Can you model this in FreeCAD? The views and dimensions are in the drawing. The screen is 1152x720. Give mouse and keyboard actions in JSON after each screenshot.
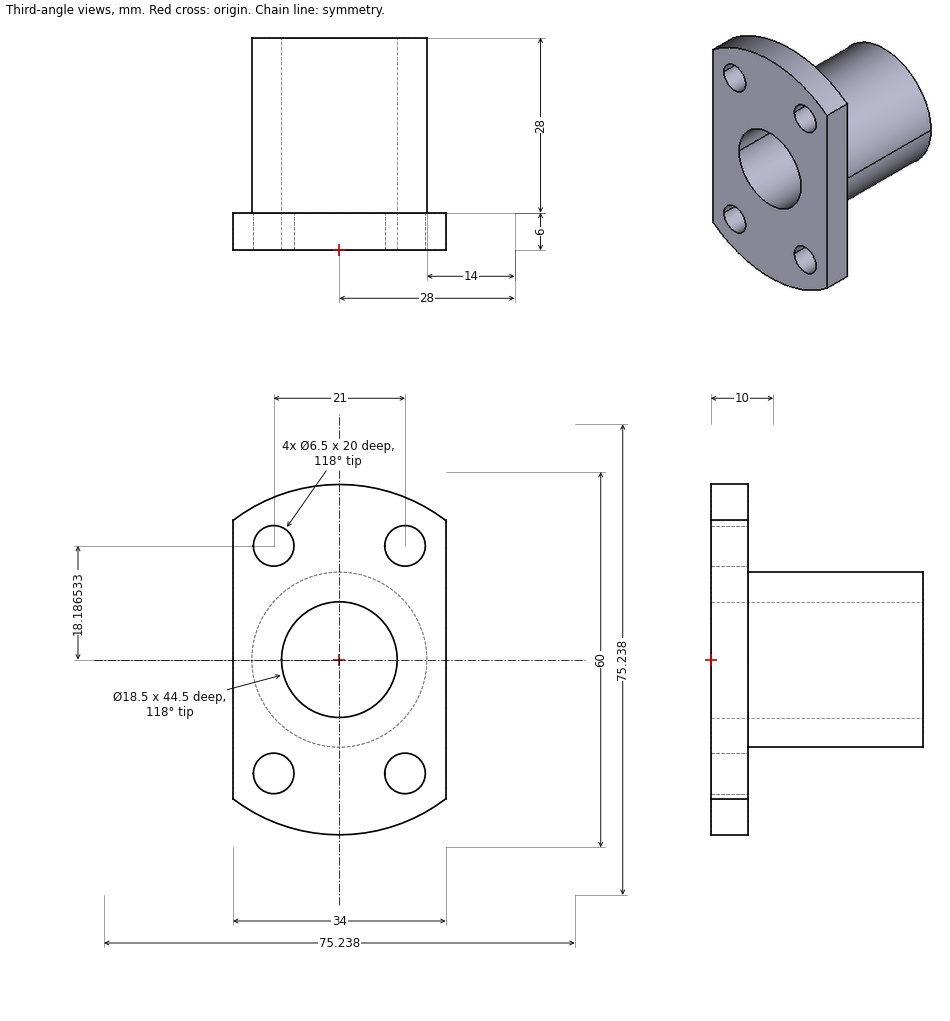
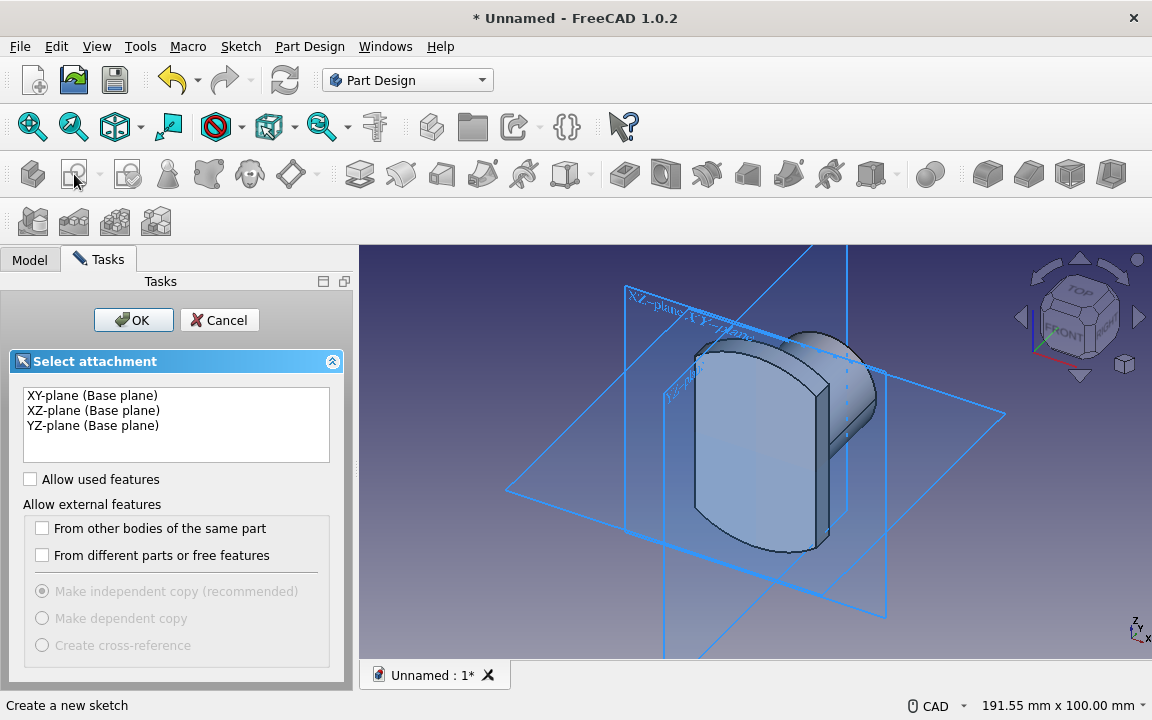
{"action": "left_click", "coordinate": [84, 410]}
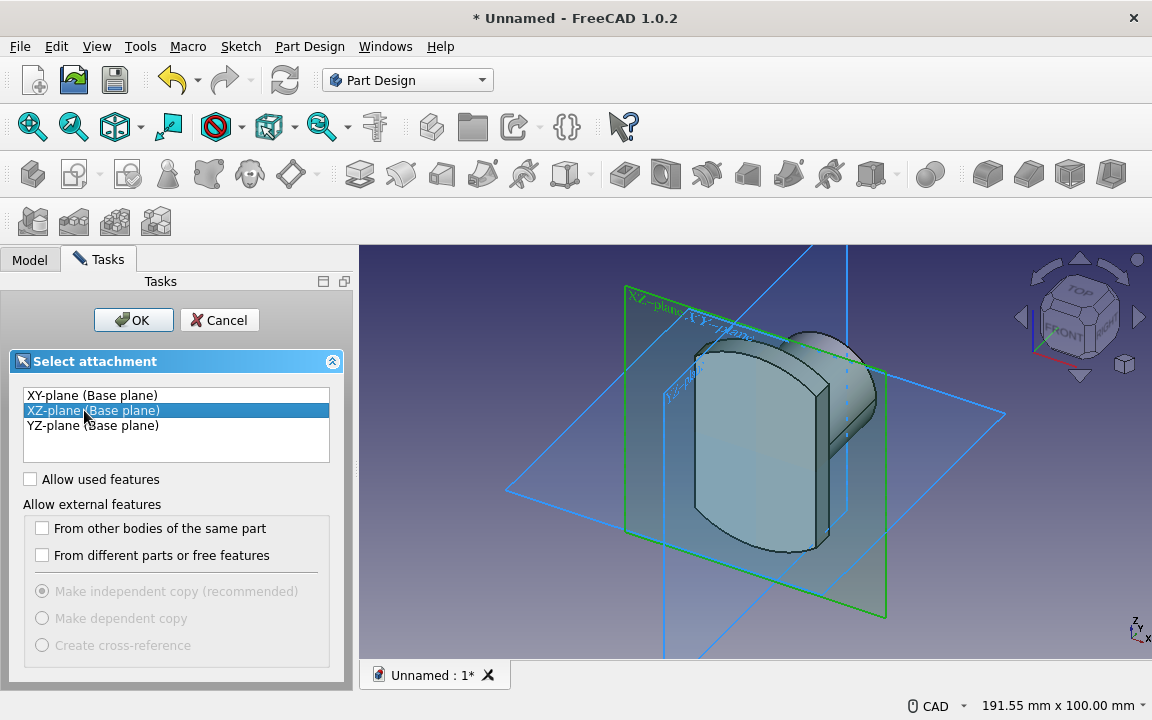
{"action": "left_click", "coordinate": [134, 320]}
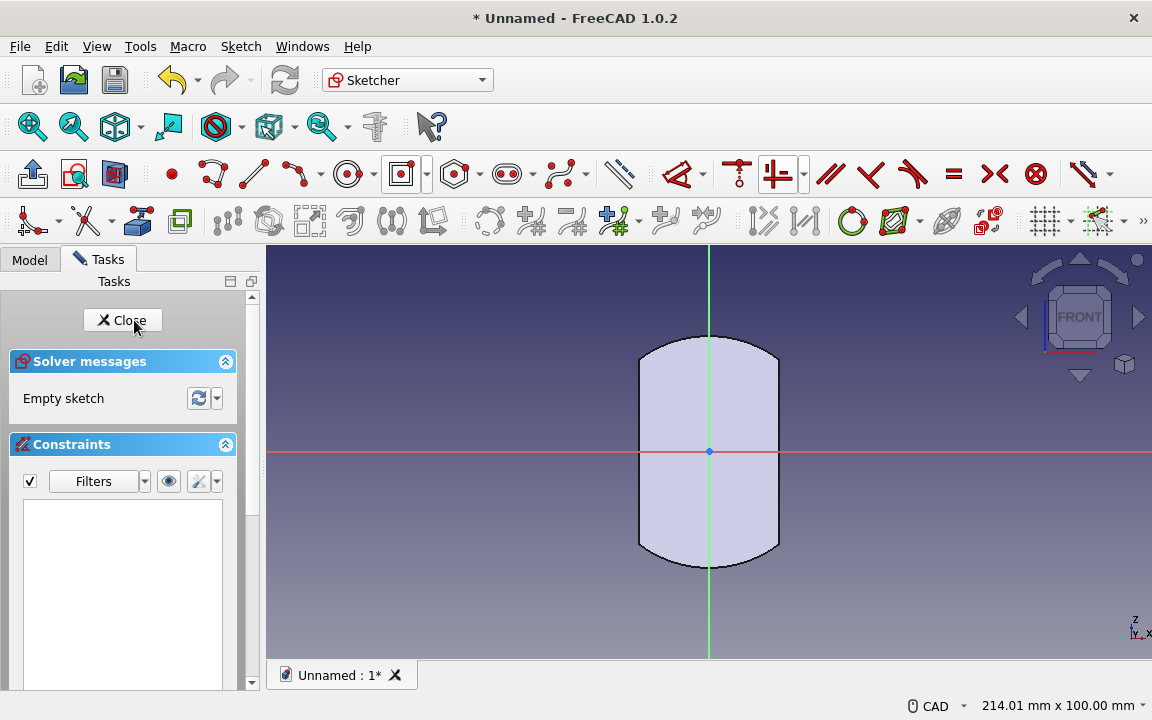
{"action": "scroll", "coordinate": [848, 452], "scroll_direction": "up", "scroll_amount": 2}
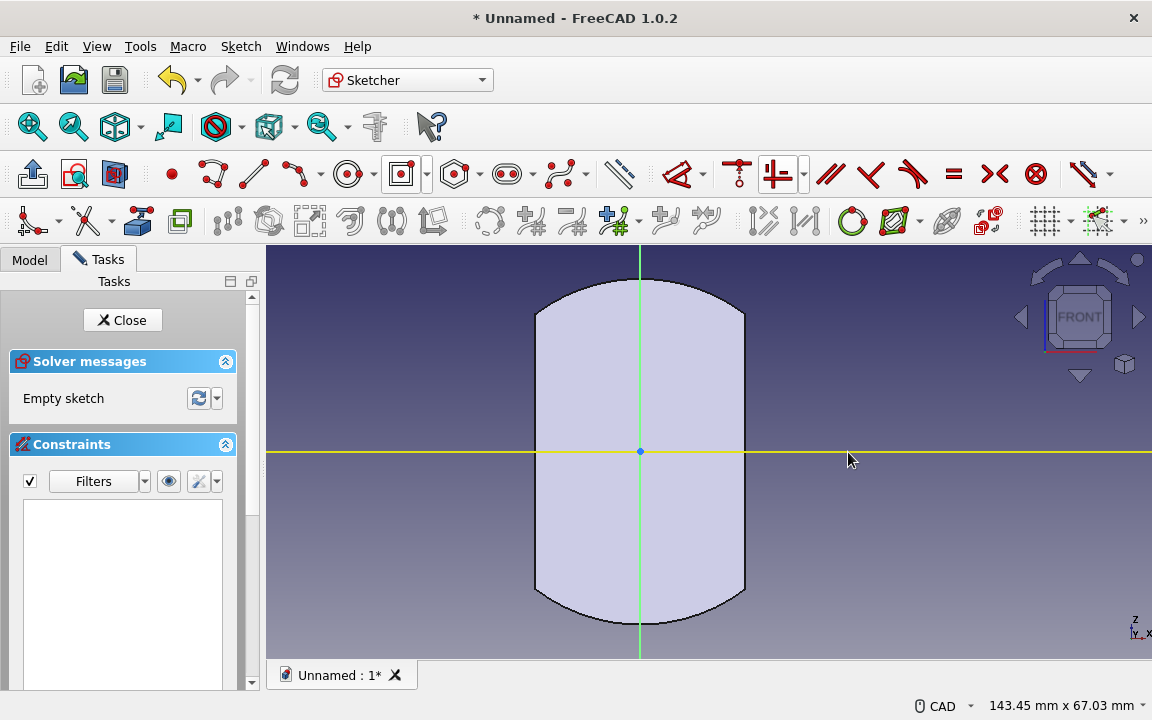
{"action": "left_click", "coordinate": [348, 174]}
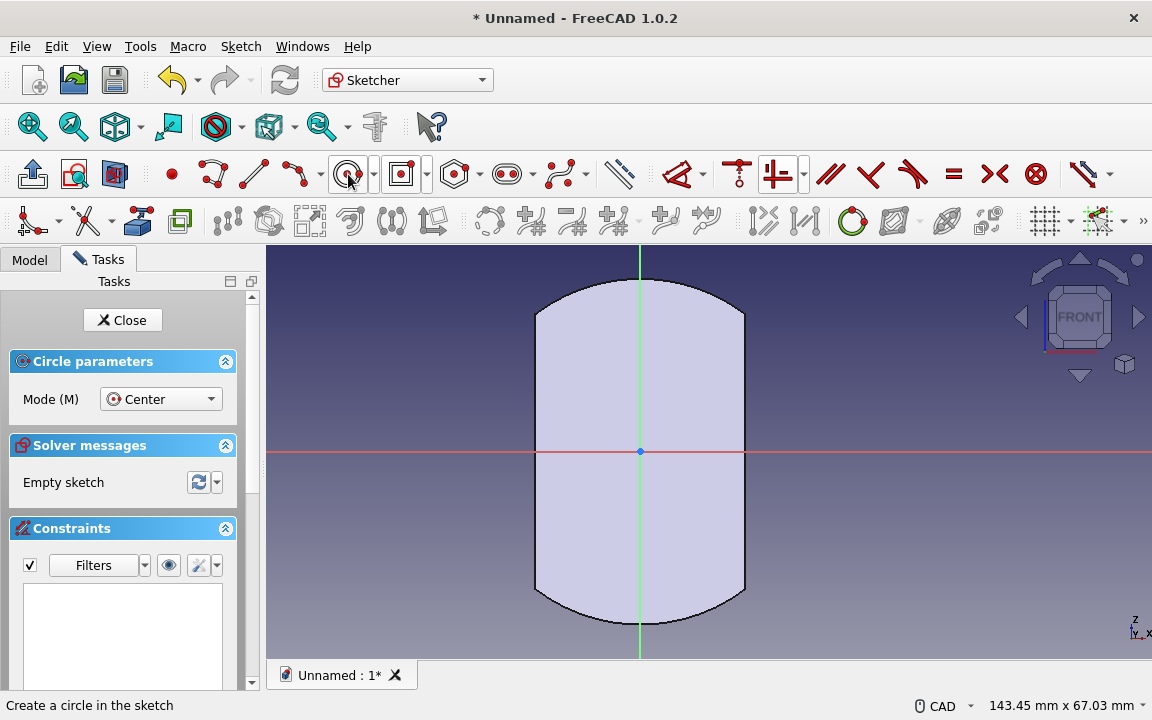
{"action": "left_click", "coordinate": [575, 339]}
{"action": "mouse_move", "coordinate": [590, 325]}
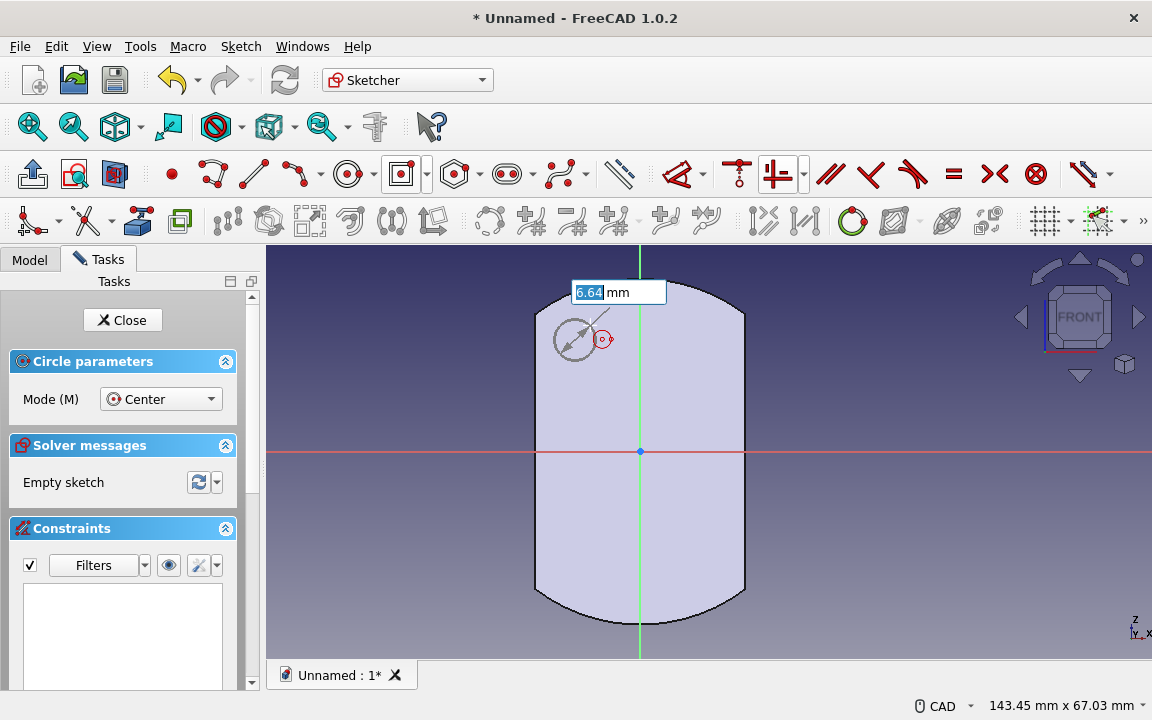
{"action": "type", "text": "6.5"}
{"action": "key", "text": "Return"}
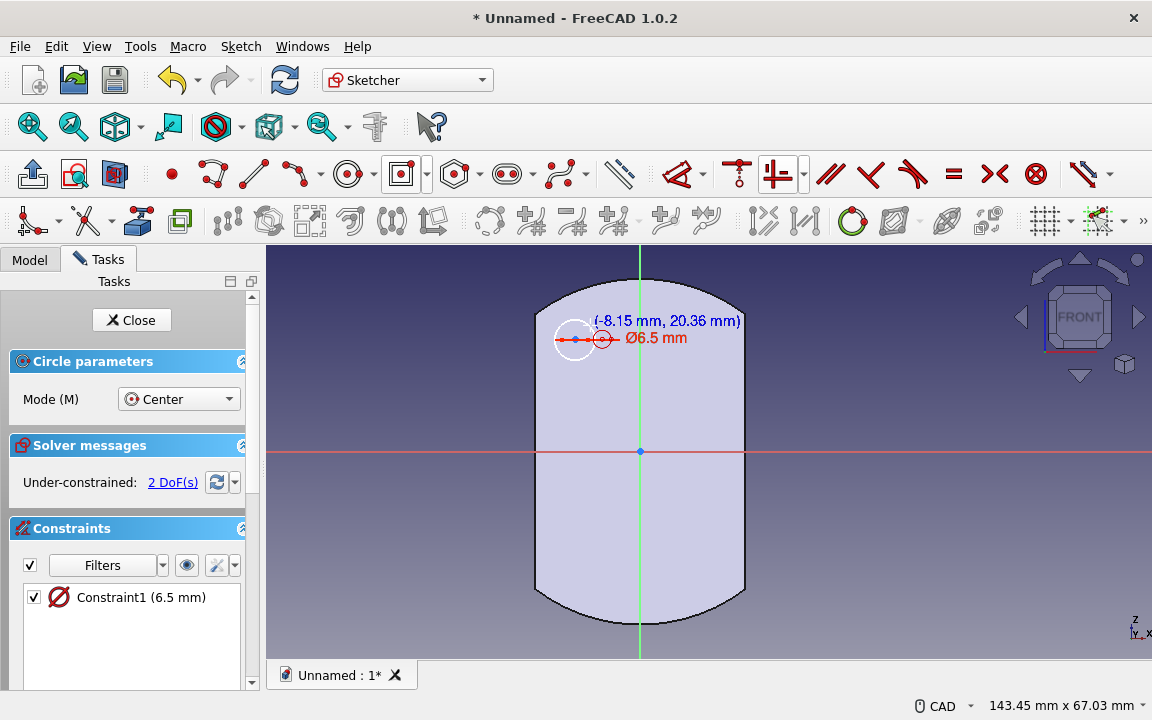
{"action": "left_click", "coordinate": [705, 339]}
{"action": "mouse_move", "coordinate": [719, 325]}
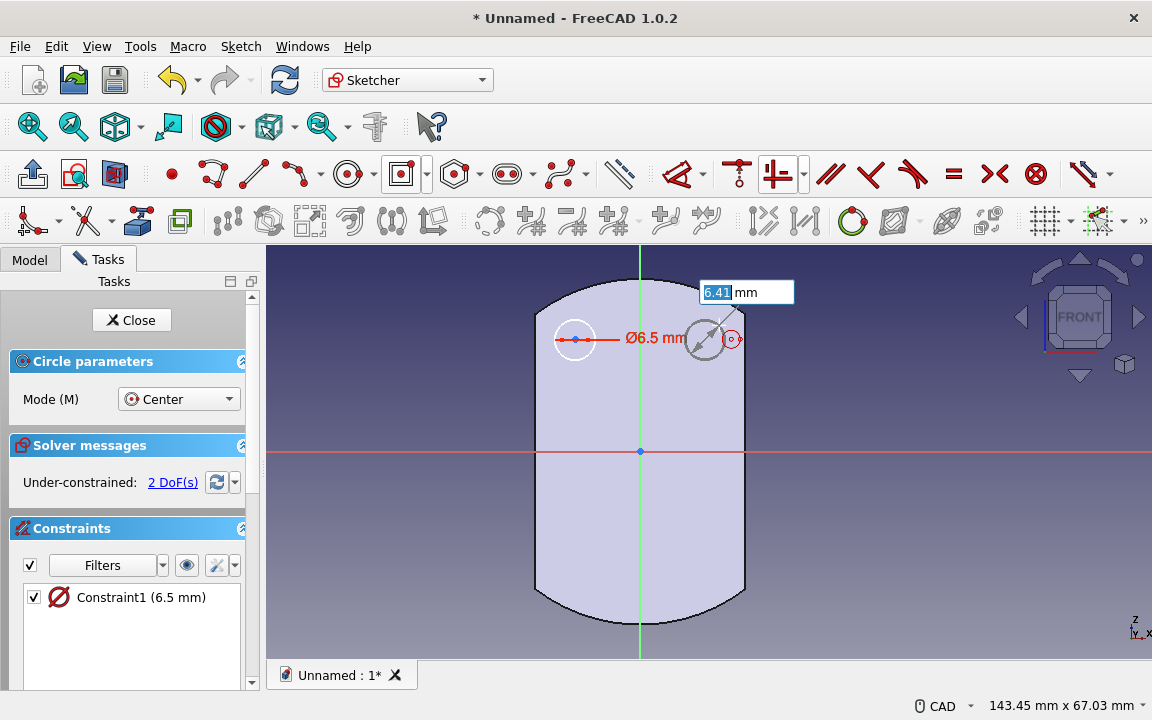
{"action": "type", "text": "6.5"}
{"action": "key", "text": "Return"}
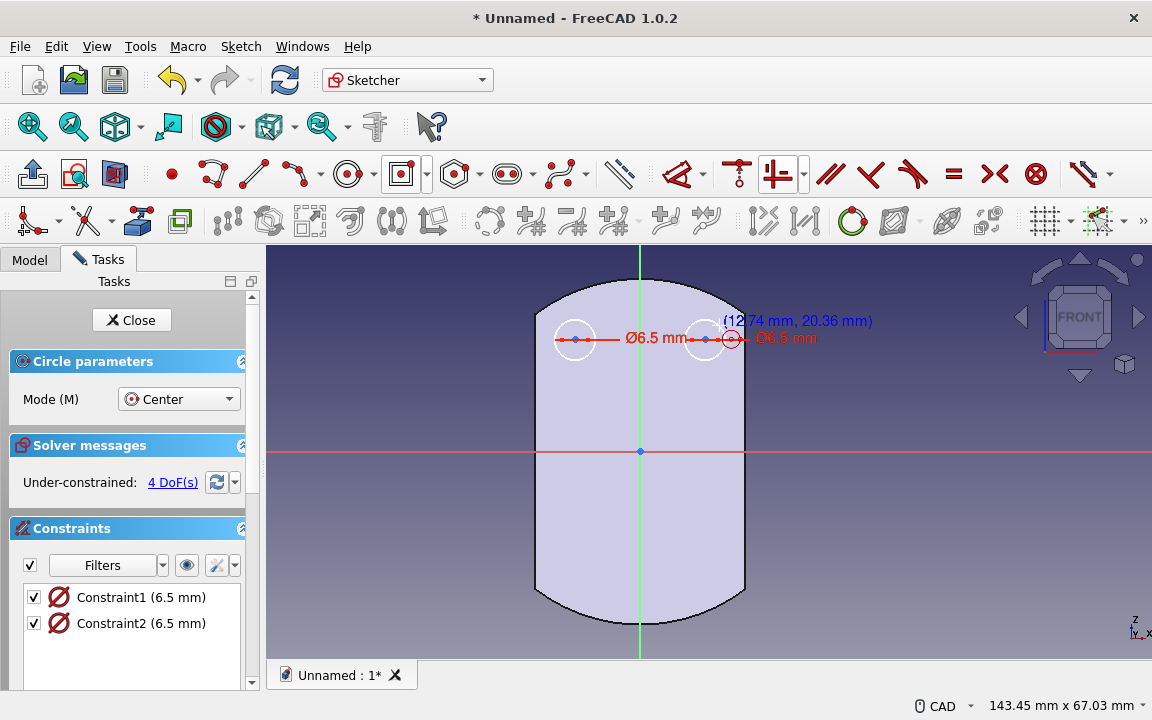
{"action": "left_click", "coordinate": [575, 564]}
{"action": "mouse_move", "coordinate": [590, 550]}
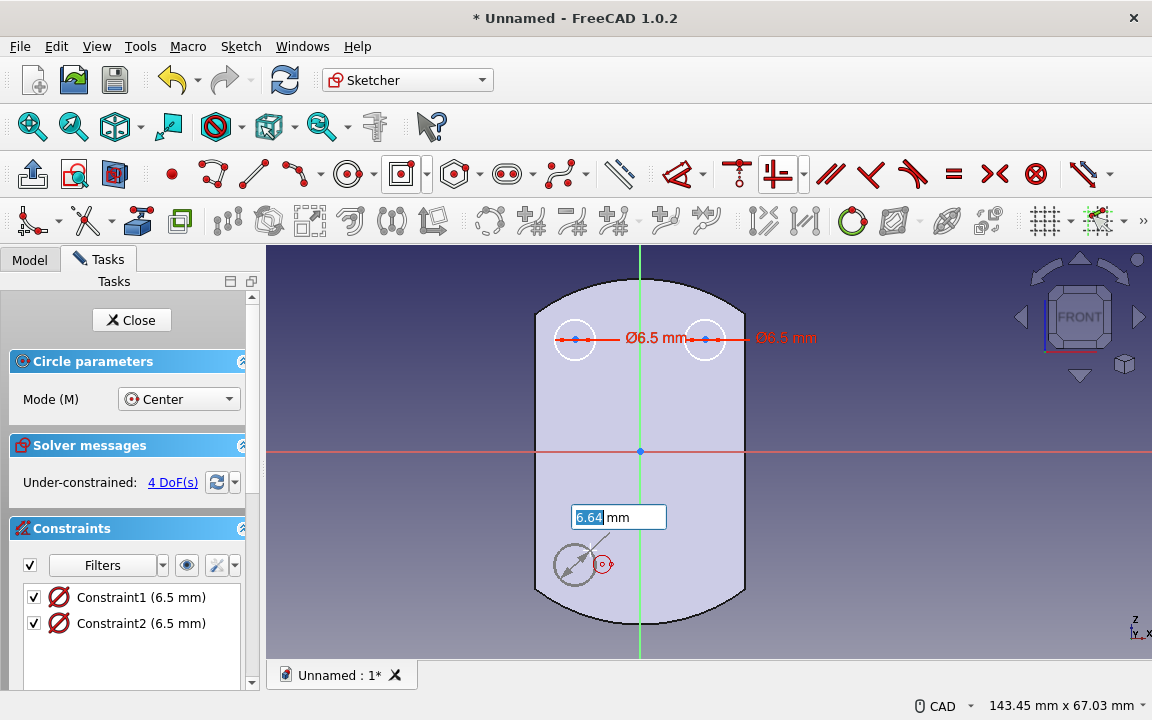
{"action": "type", "text": "6.5"}
{"action": "key", "text": "Return"}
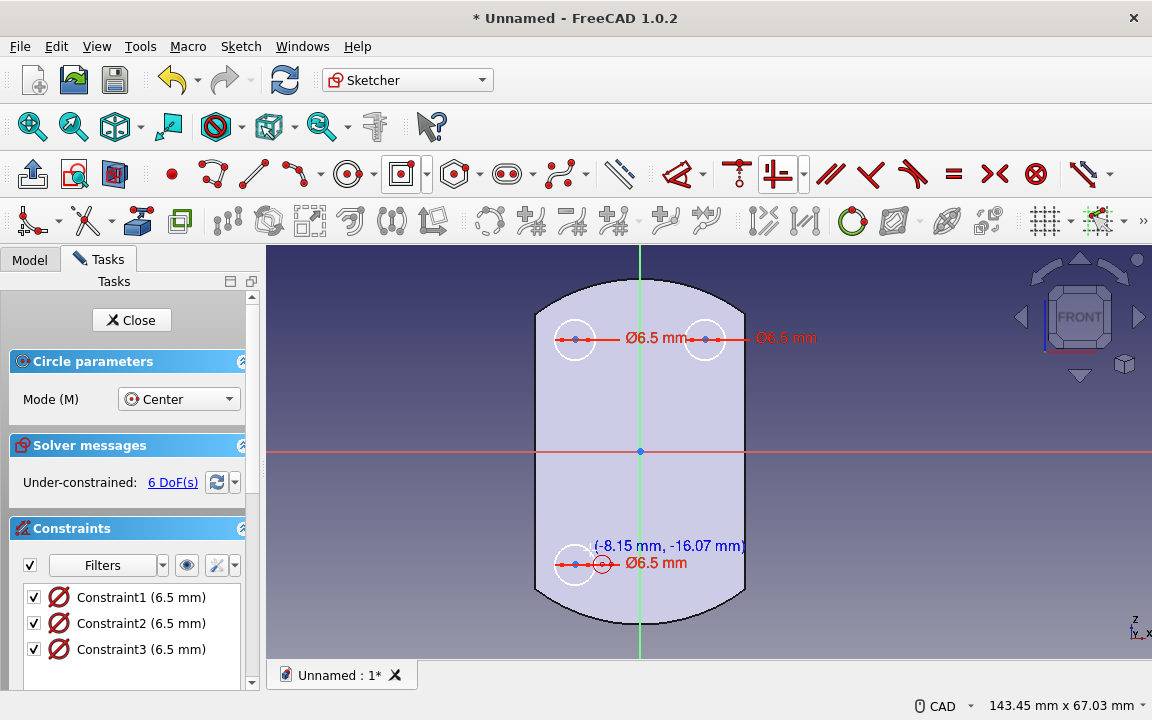
{"action": "left_click", "coordinate": [705, 564]}
{"action": "mouse_move", "coordinate": [719, 550]}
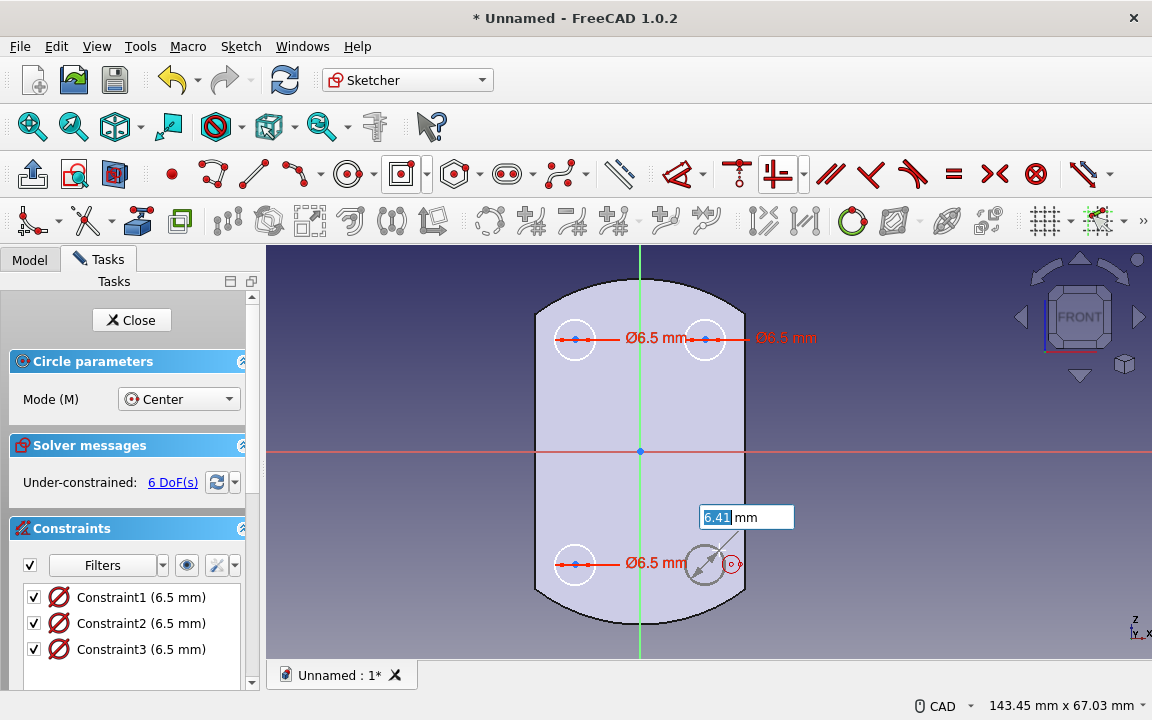
{"action": "type", "text": "6.5"}
{"action": "key", "text": "Return"}
{"action": "key", "text": "Escape"}